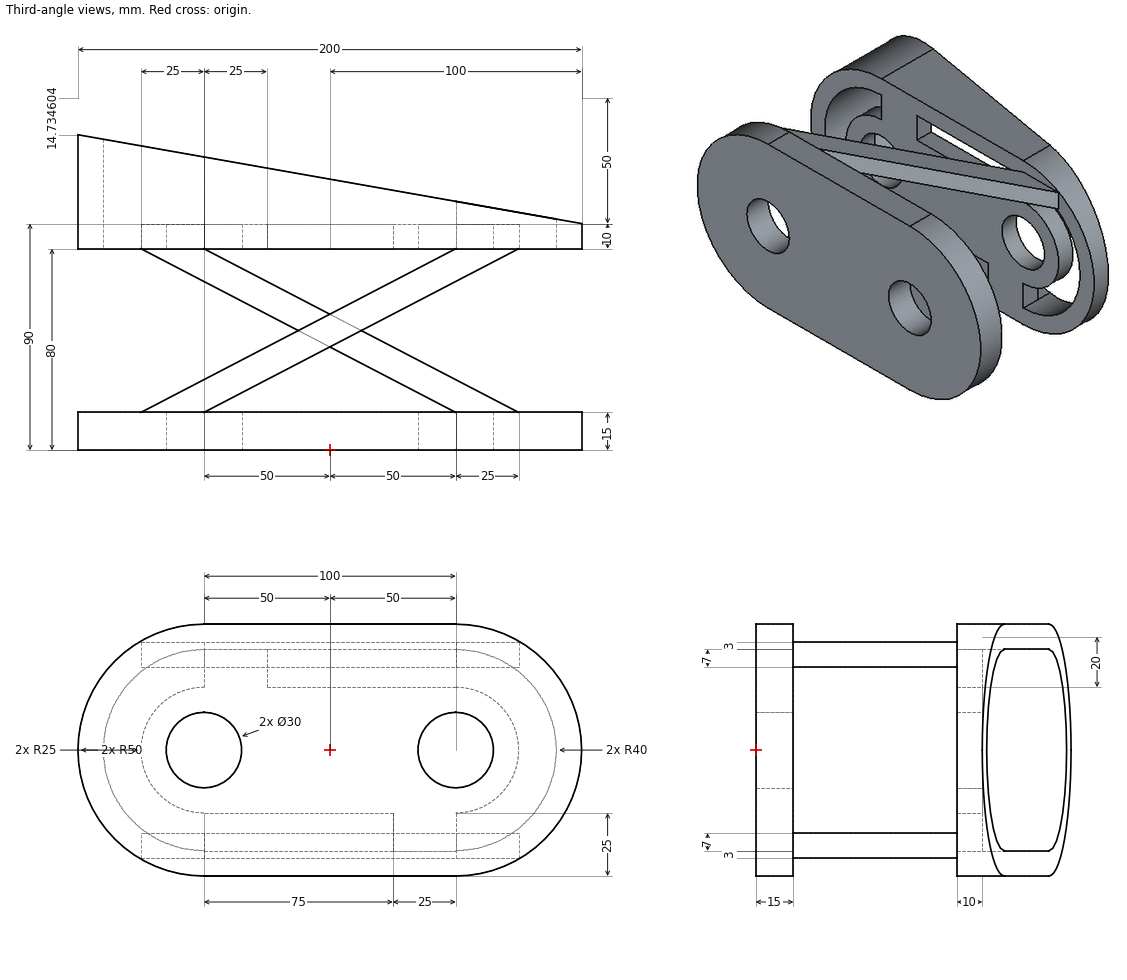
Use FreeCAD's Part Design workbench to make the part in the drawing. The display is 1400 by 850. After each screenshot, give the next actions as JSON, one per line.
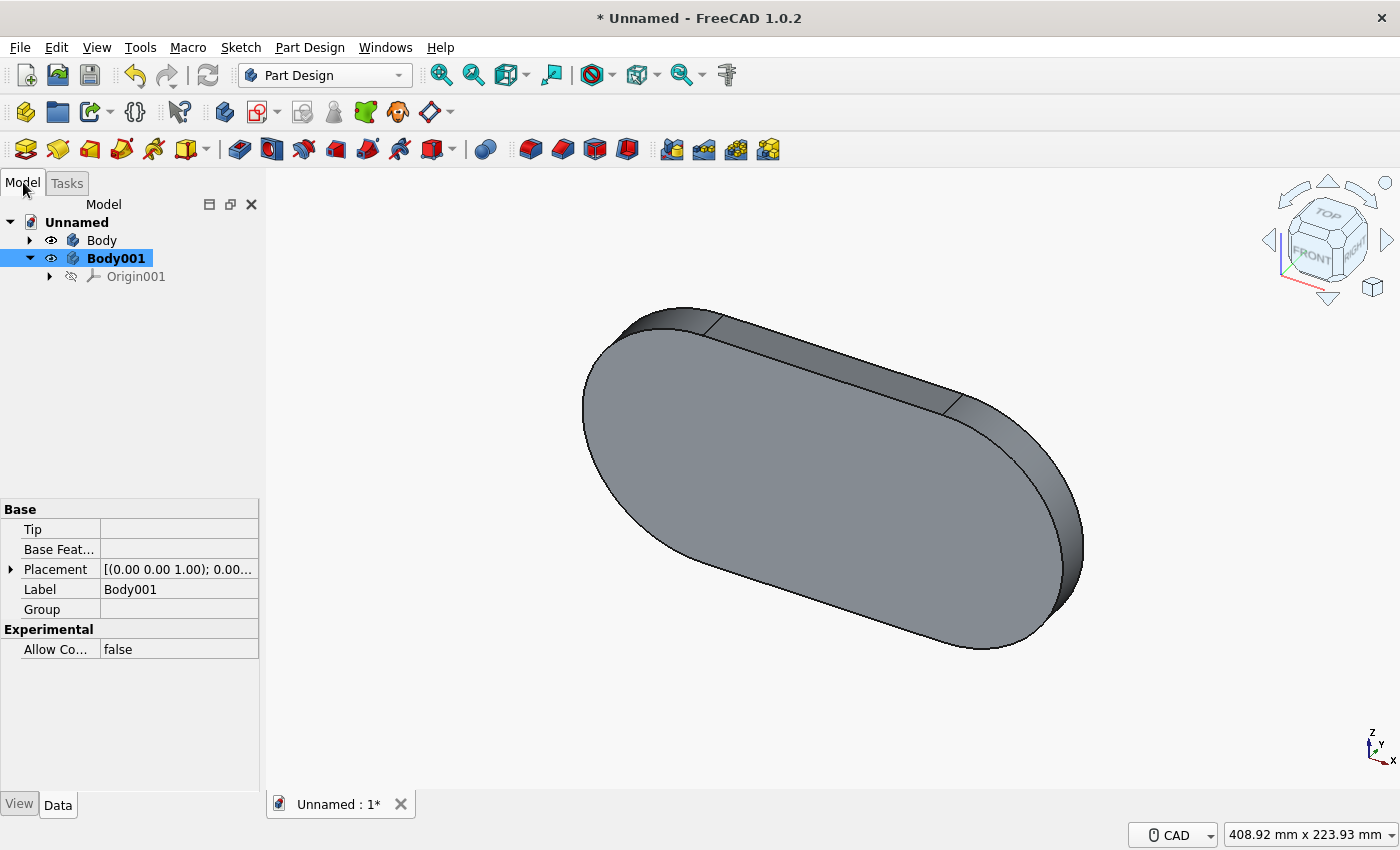
{"action": "left_click", "coordinate": [50, 276]}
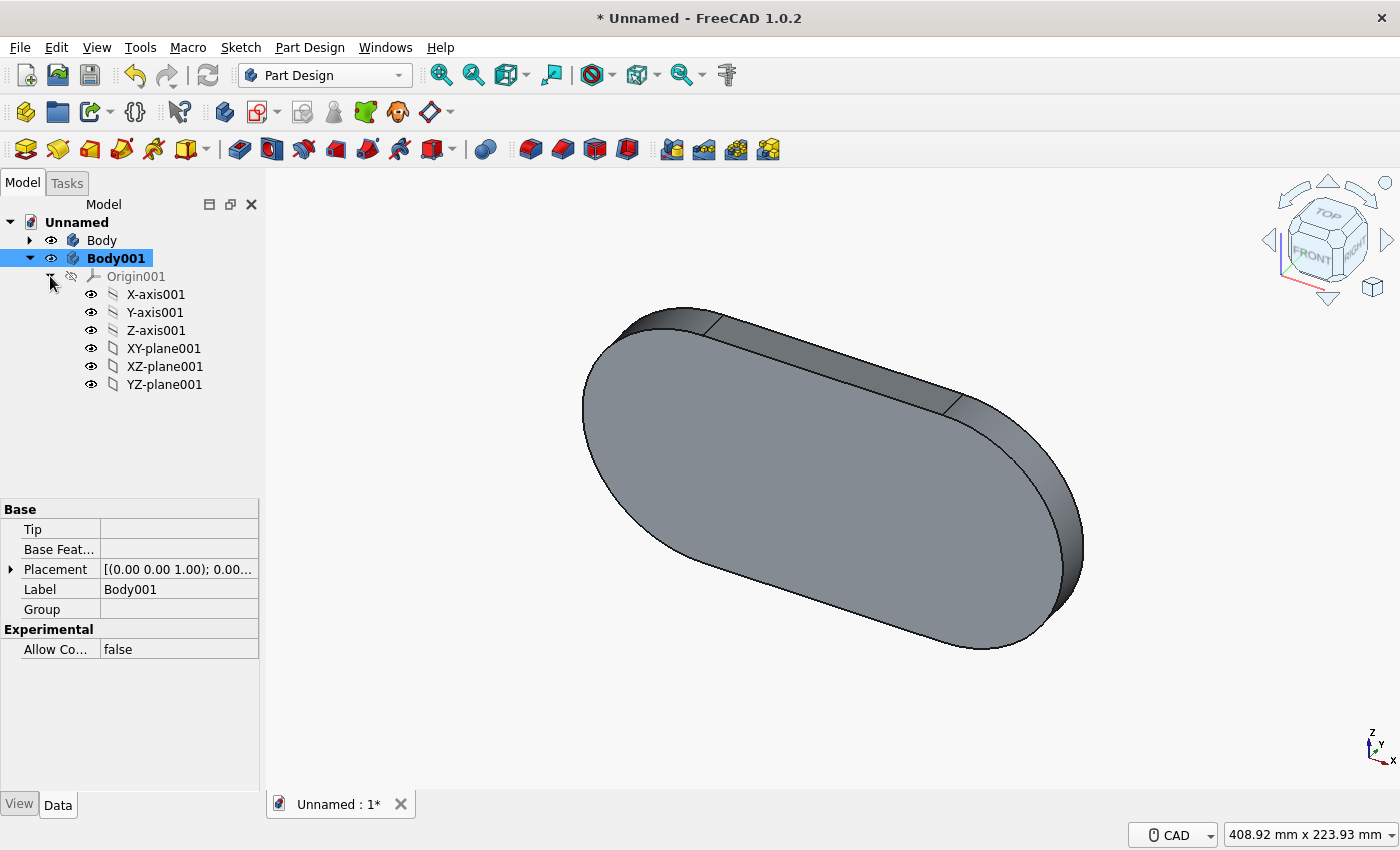
{"action": "left_click", "coordinate": [136, 366]}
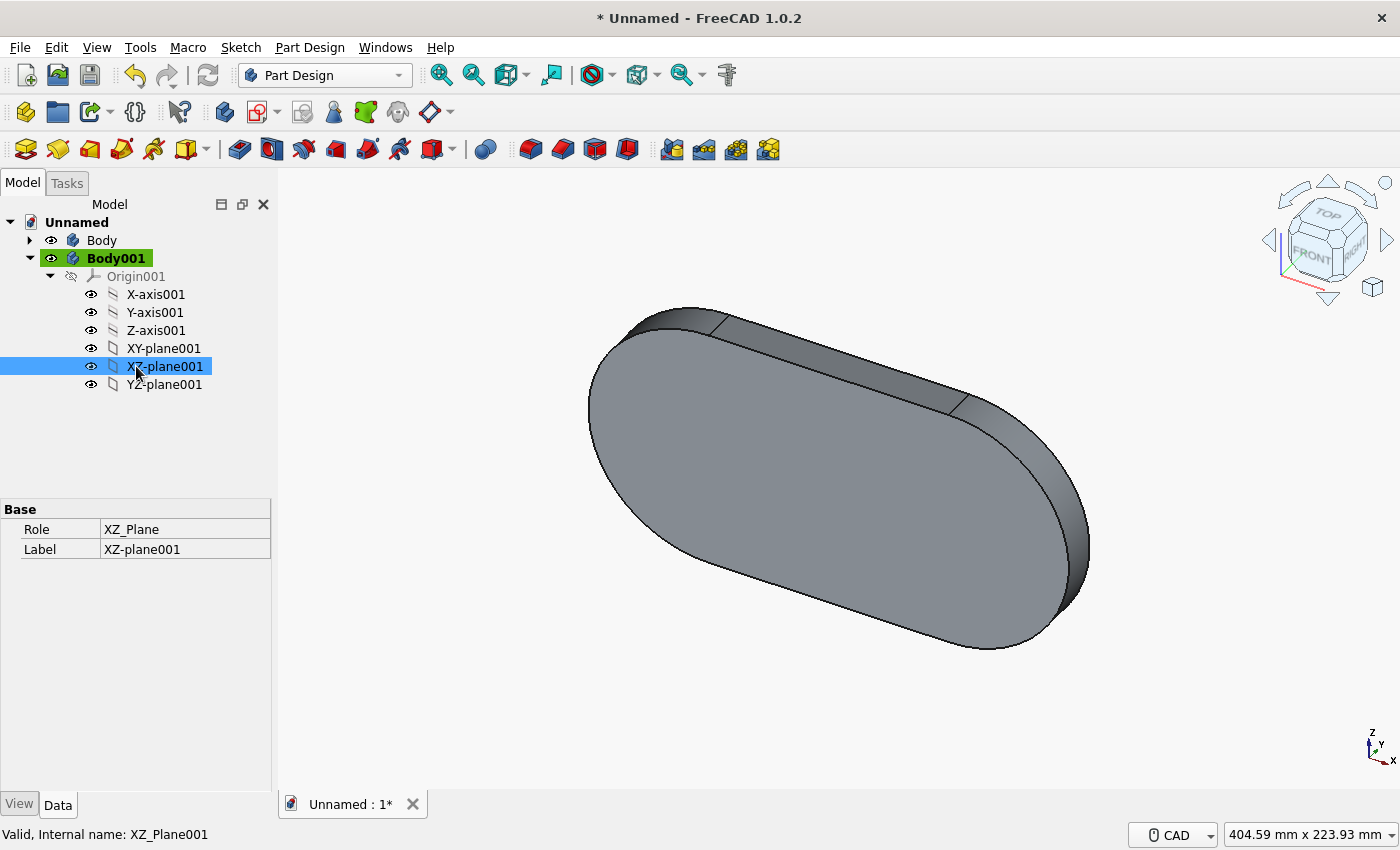
{"action": "left_click", "coordinate": [430, 112]}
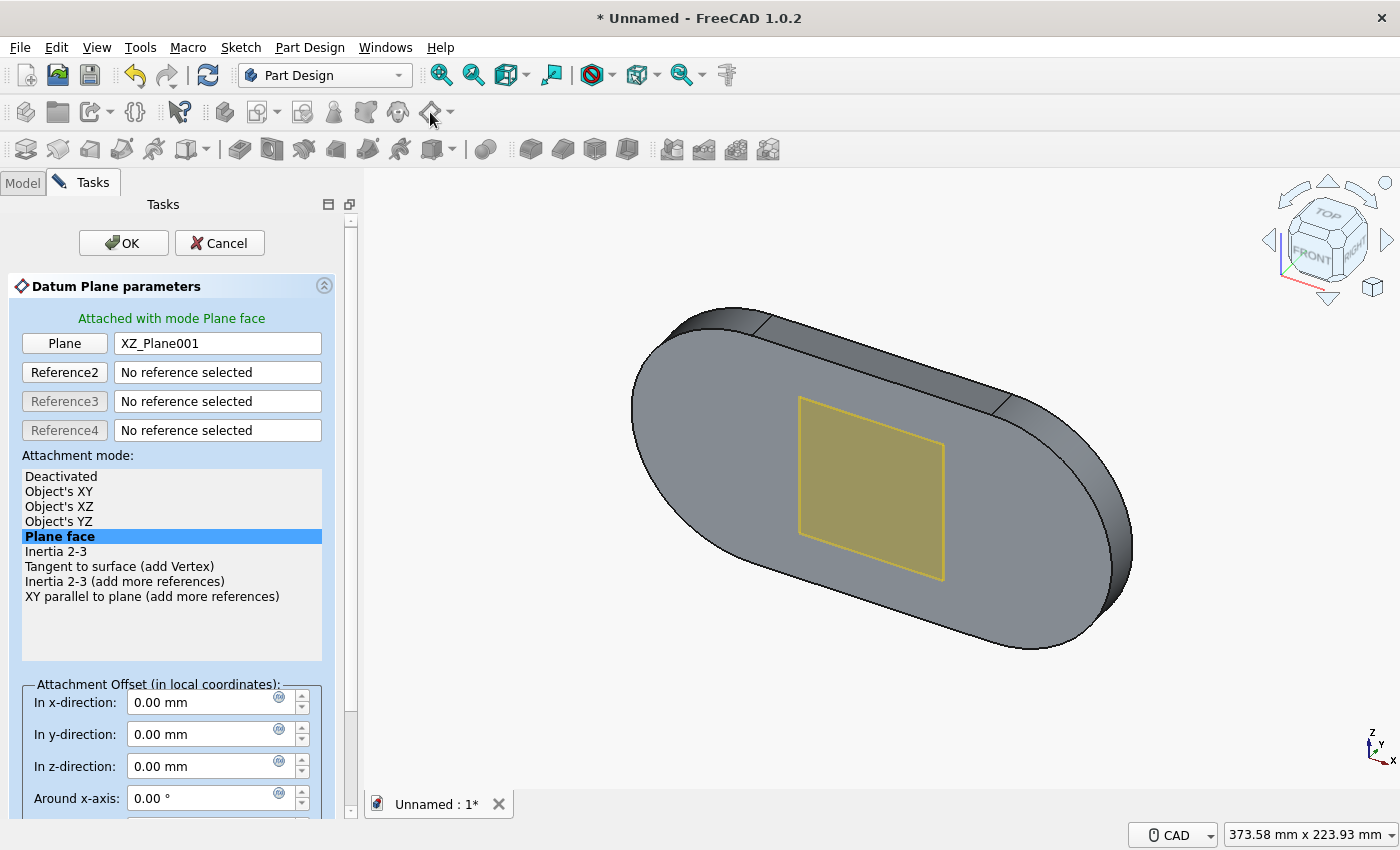
{"action": "triple_click", "coordinate": [210, 766]}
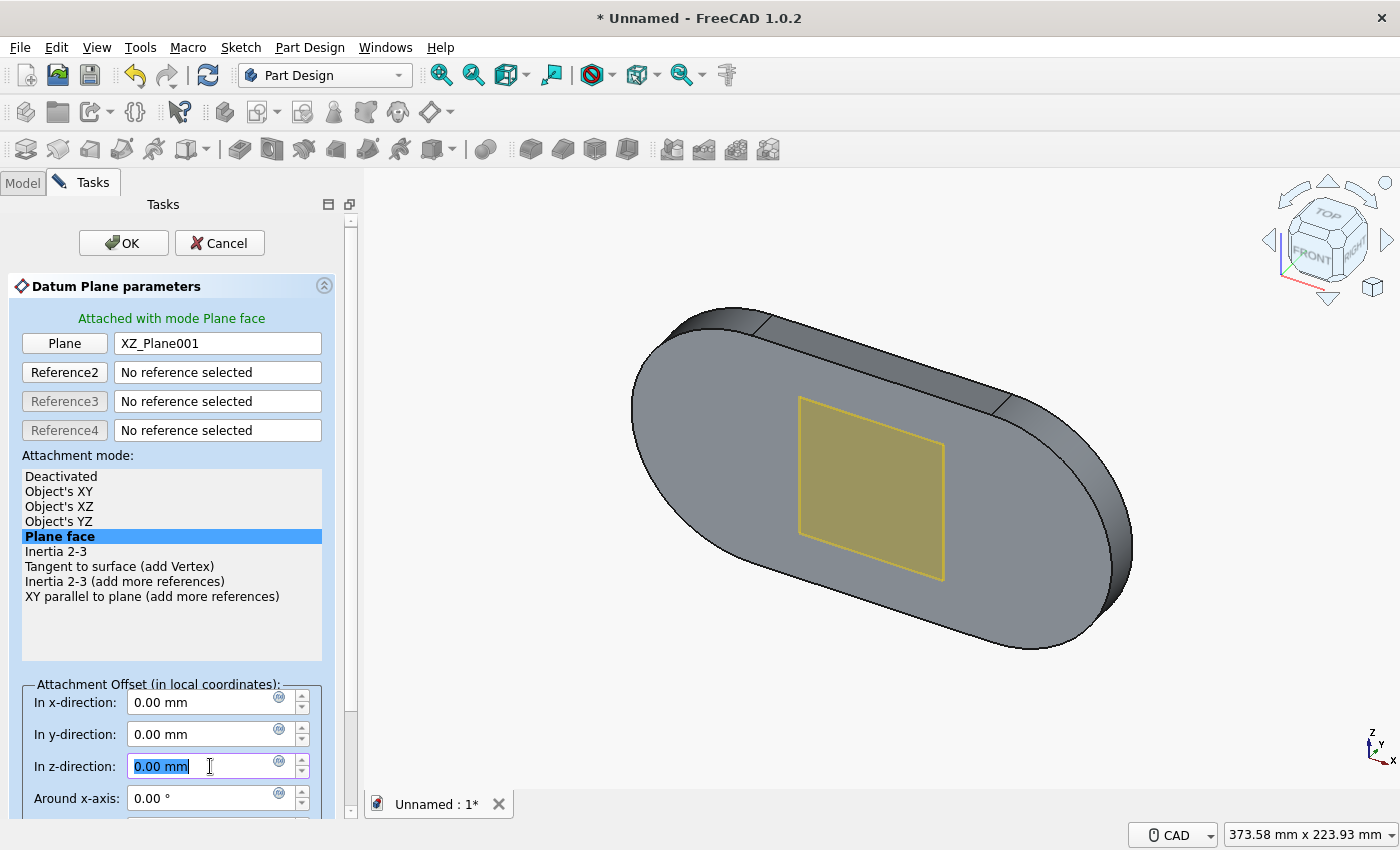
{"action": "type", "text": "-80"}
{"action": "key", "text": "Tab"}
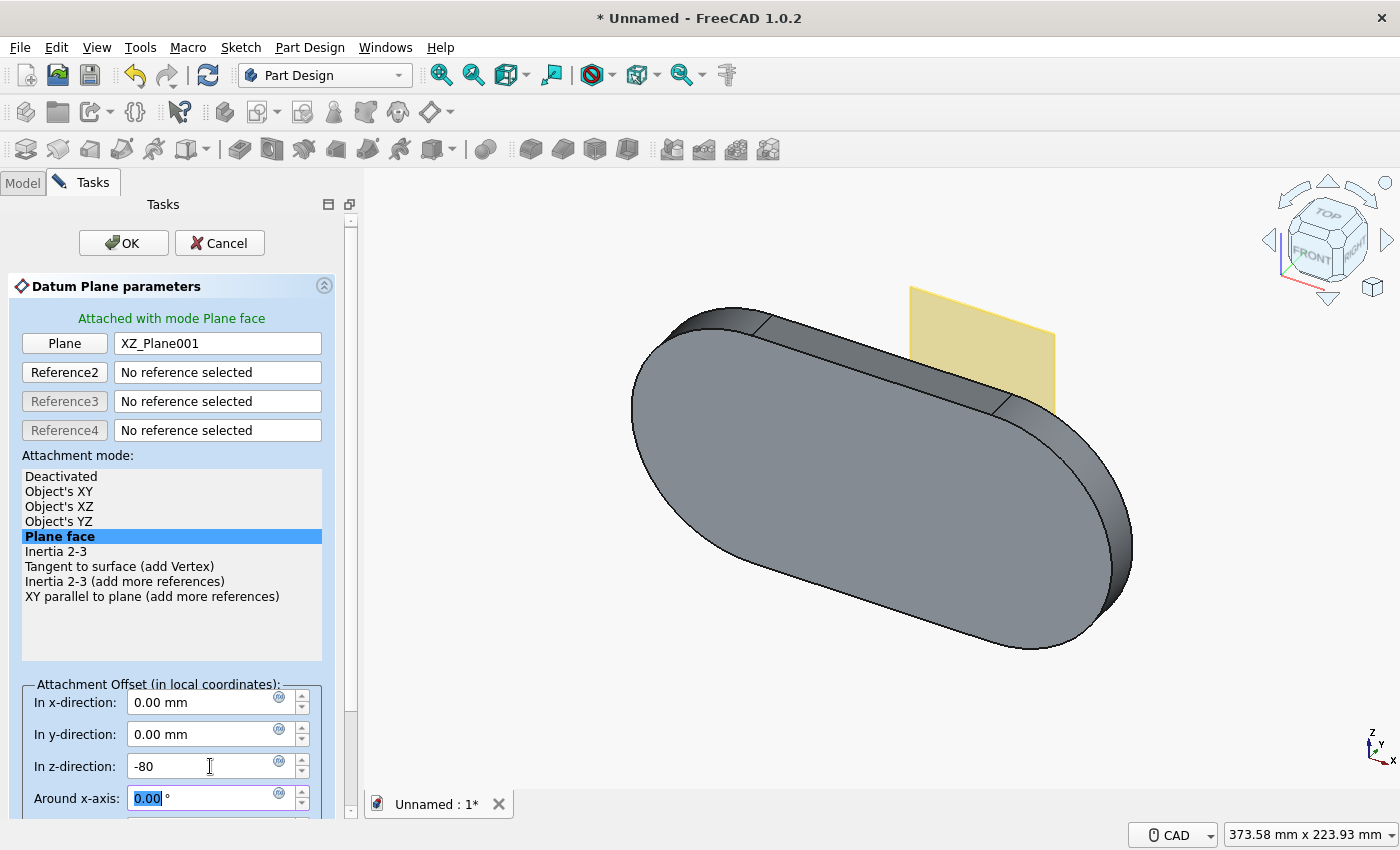
{"action": "left_click", "coordinate": [124, 243]}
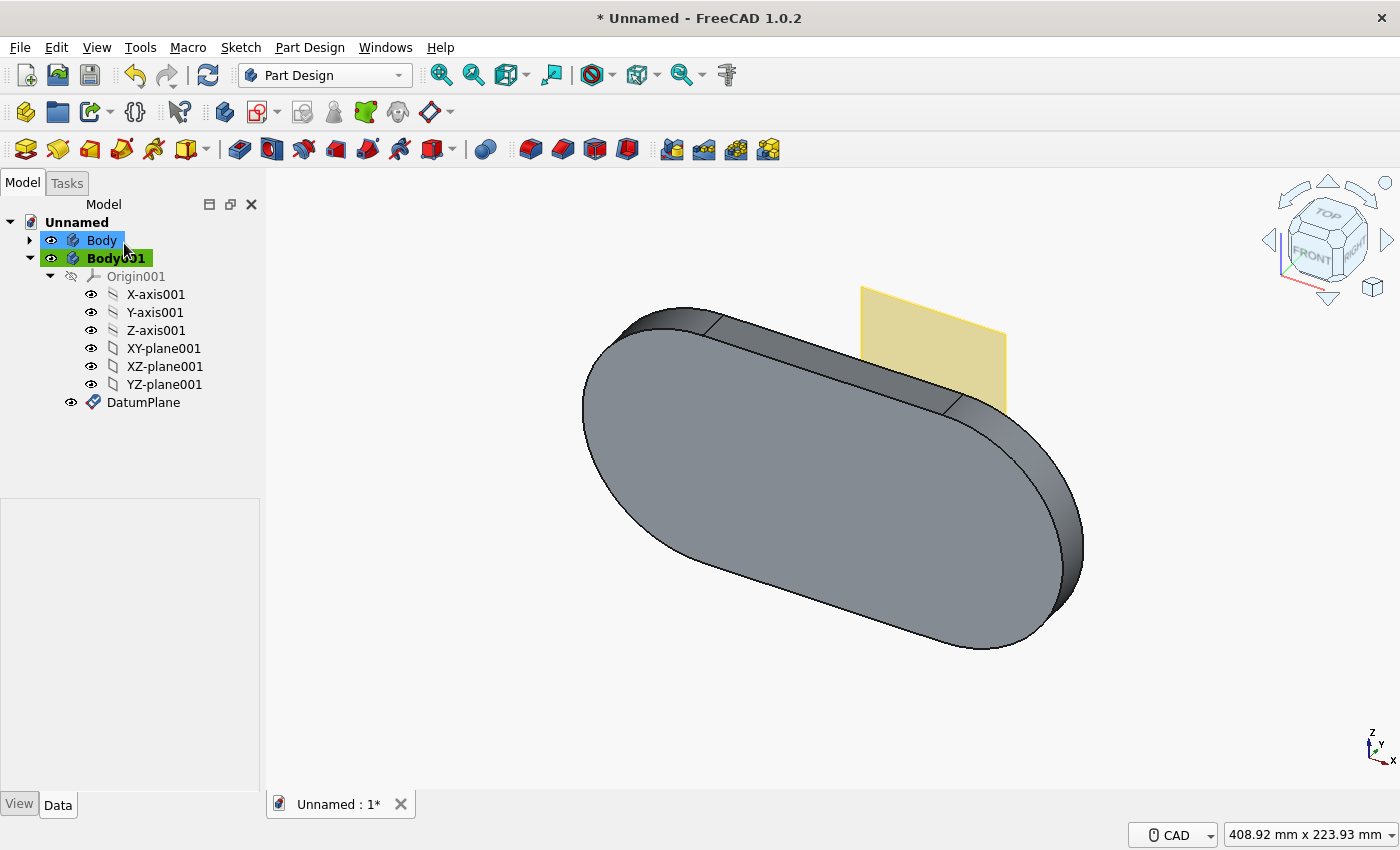
{"action": "left_click", "coordinate": [116, 402]}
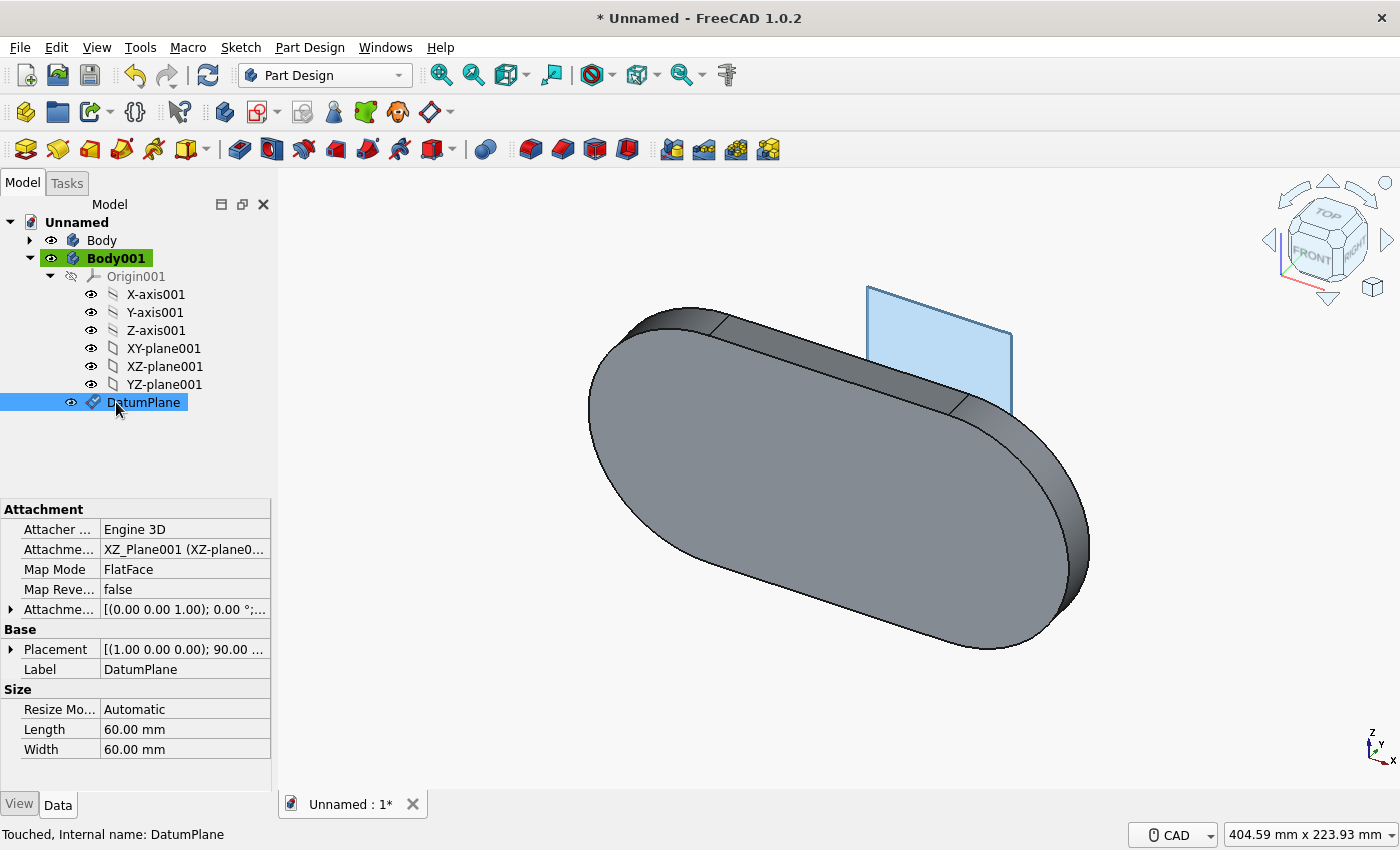
{"action": "left_click", "coordinate": [258, 112]}